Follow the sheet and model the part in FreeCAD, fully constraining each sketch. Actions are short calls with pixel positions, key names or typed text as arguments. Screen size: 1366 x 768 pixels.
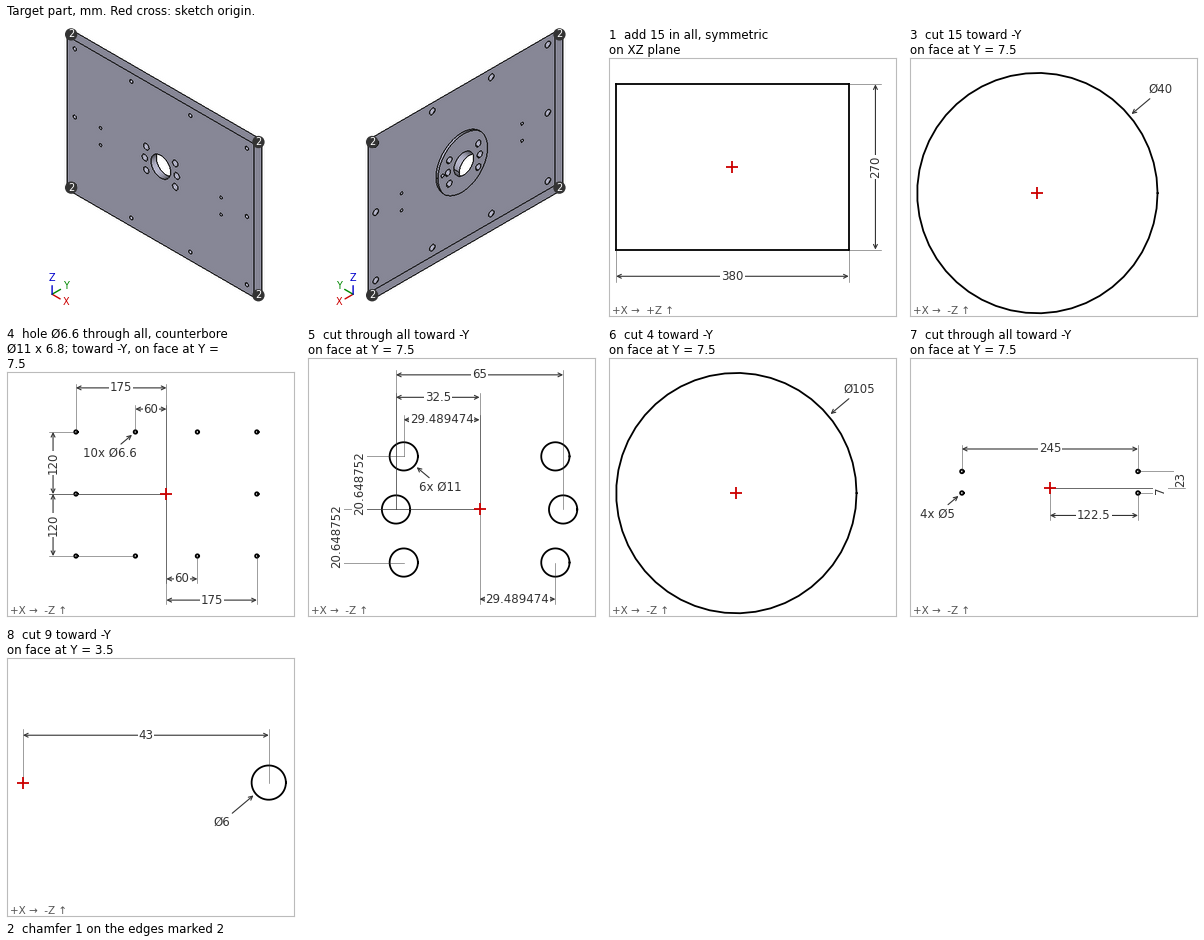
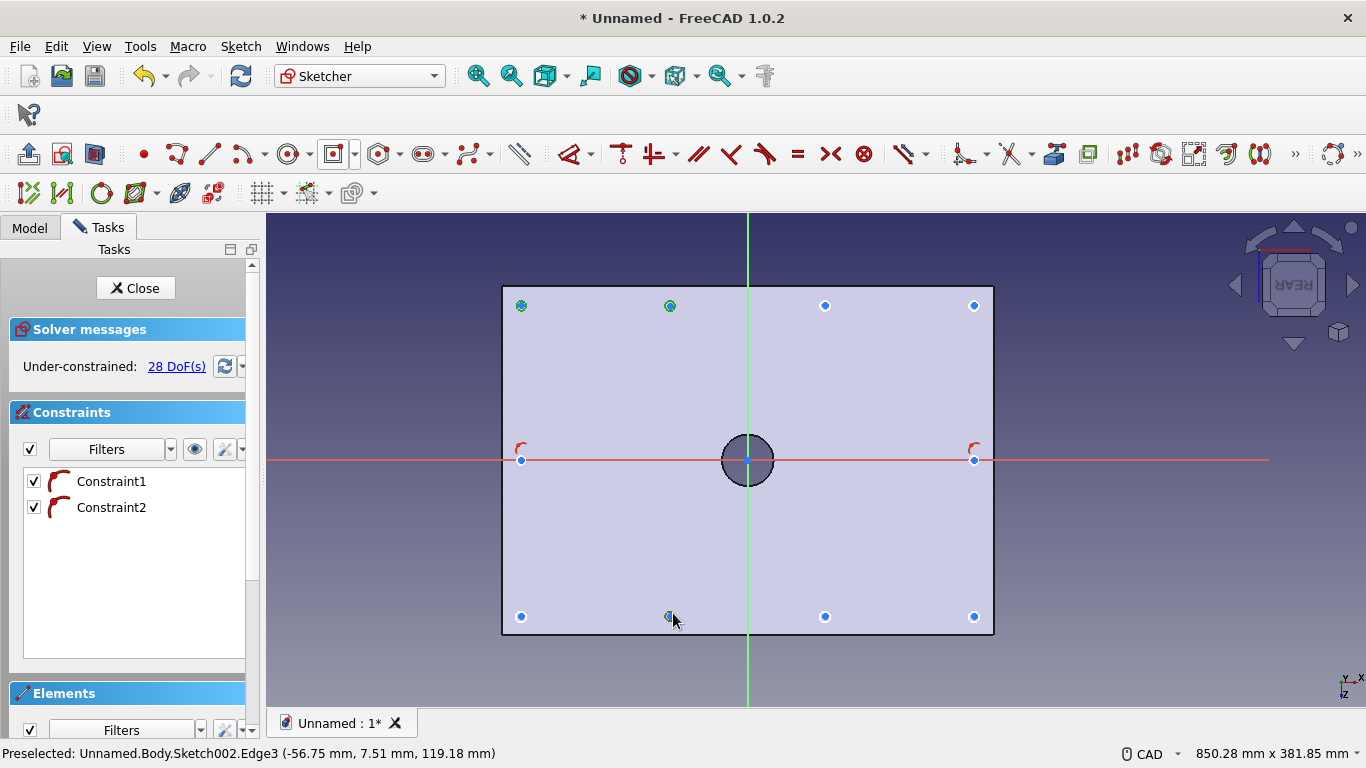
scroll(524, 457, up, 8)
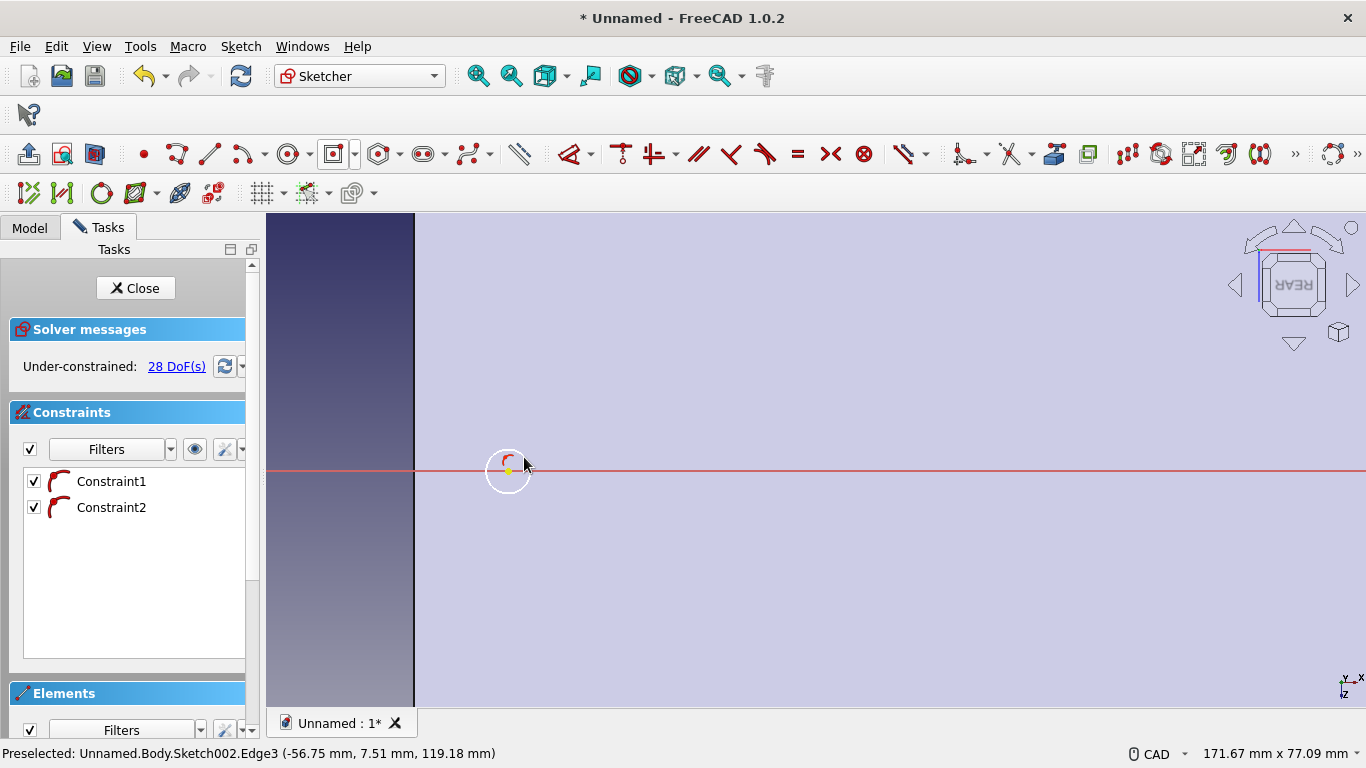
click(524, 456)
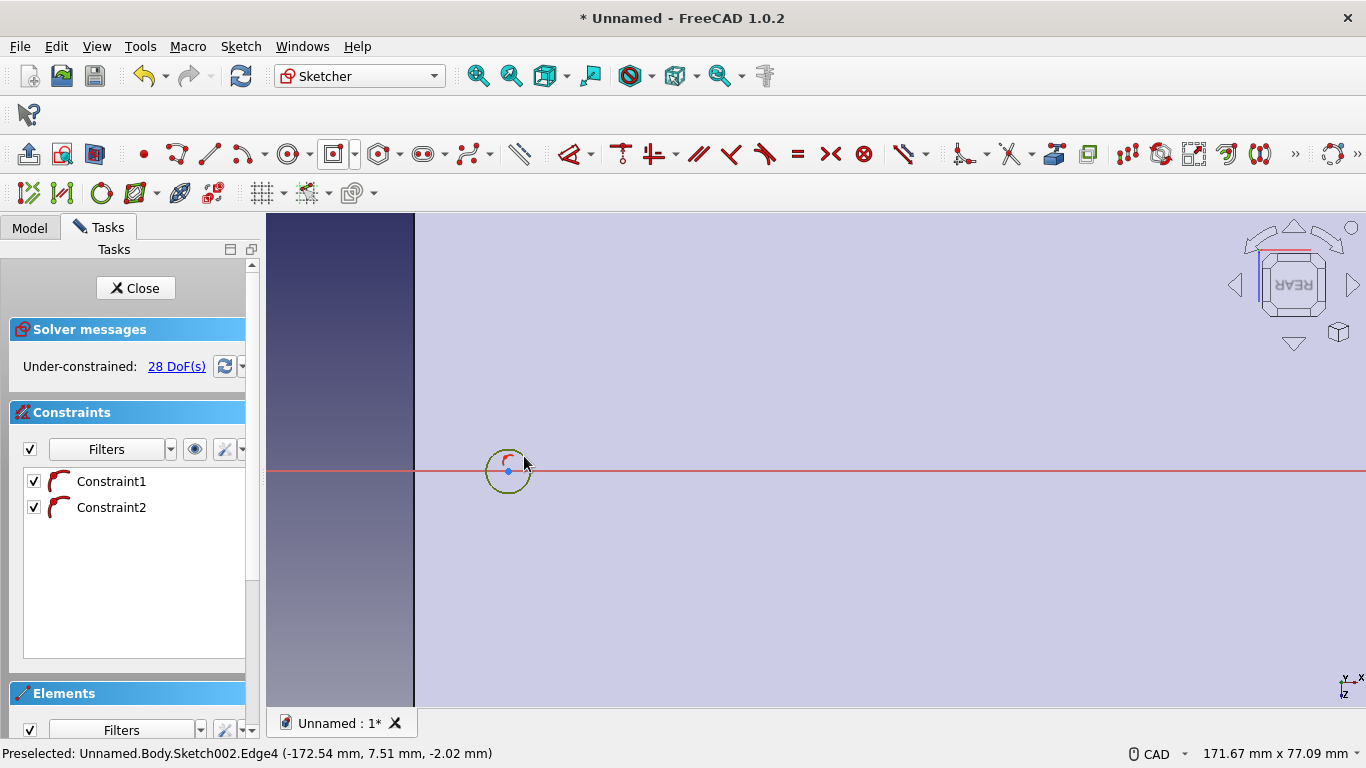
scroll(524, 457, down, 8)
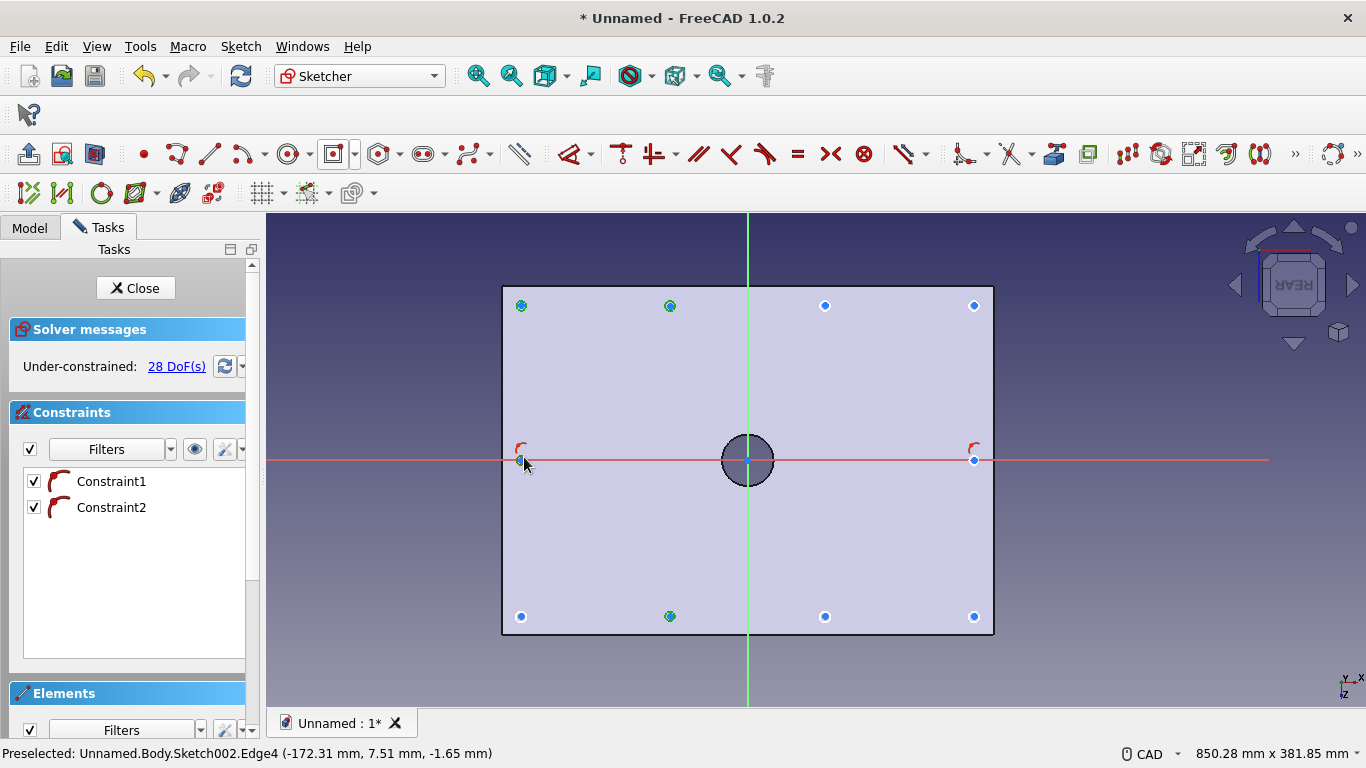
scroll(525, 613, up, 5)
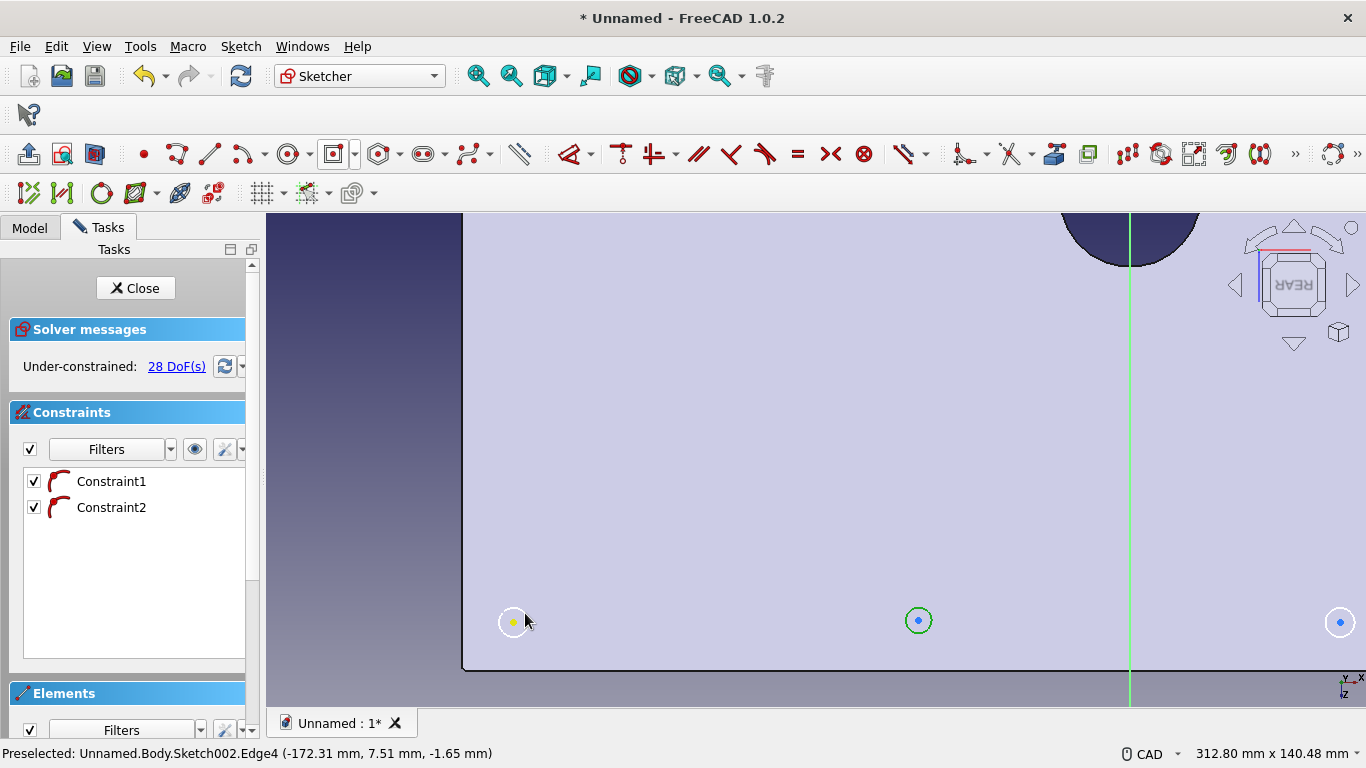
click(524, 612)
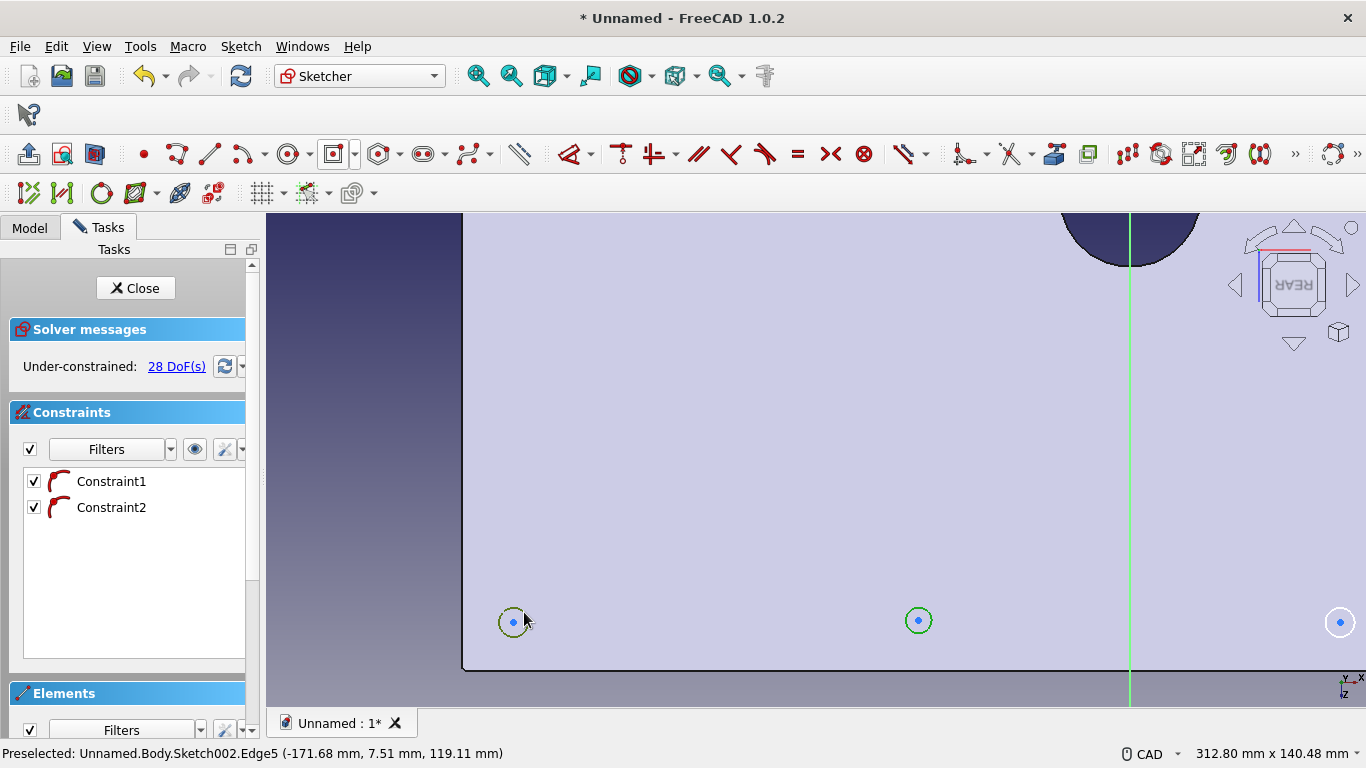
scroll(525, 613, down, 5)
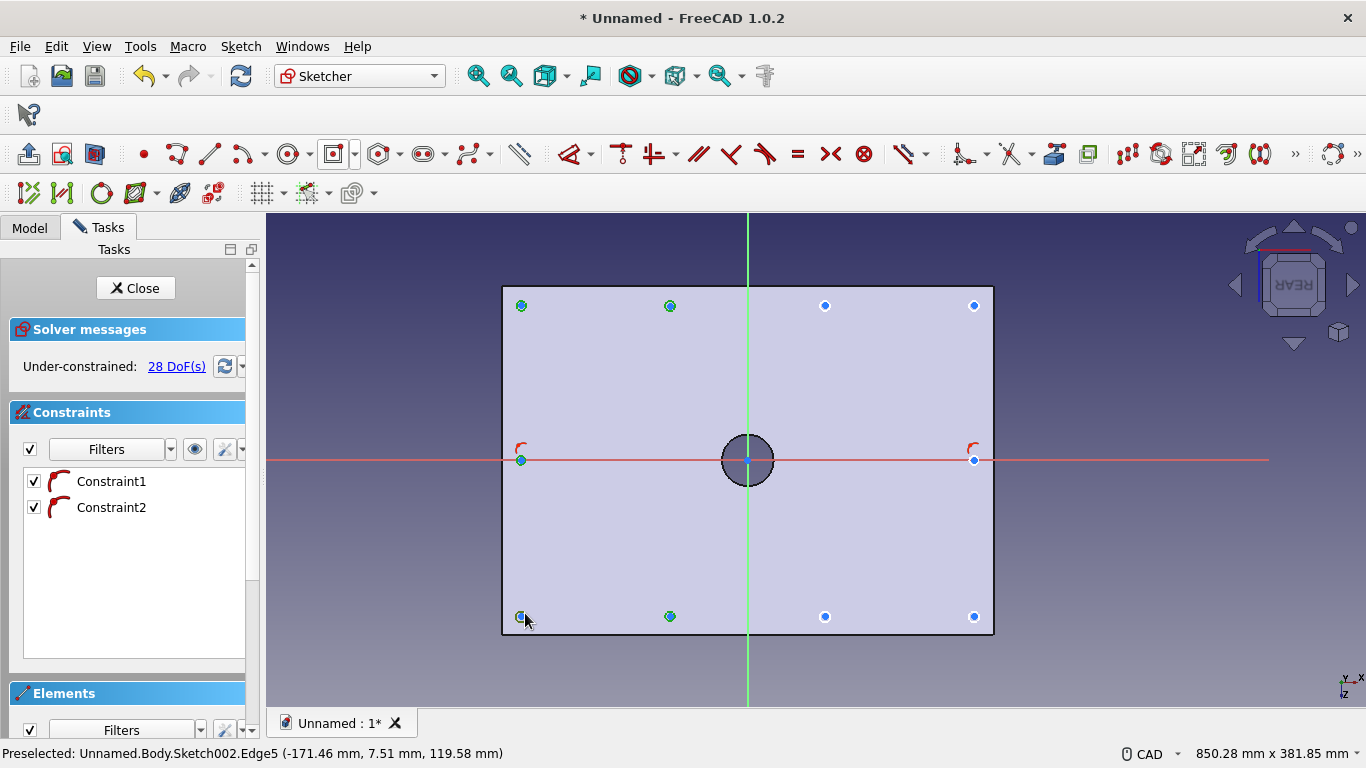
scroll(978, 613, up, 5)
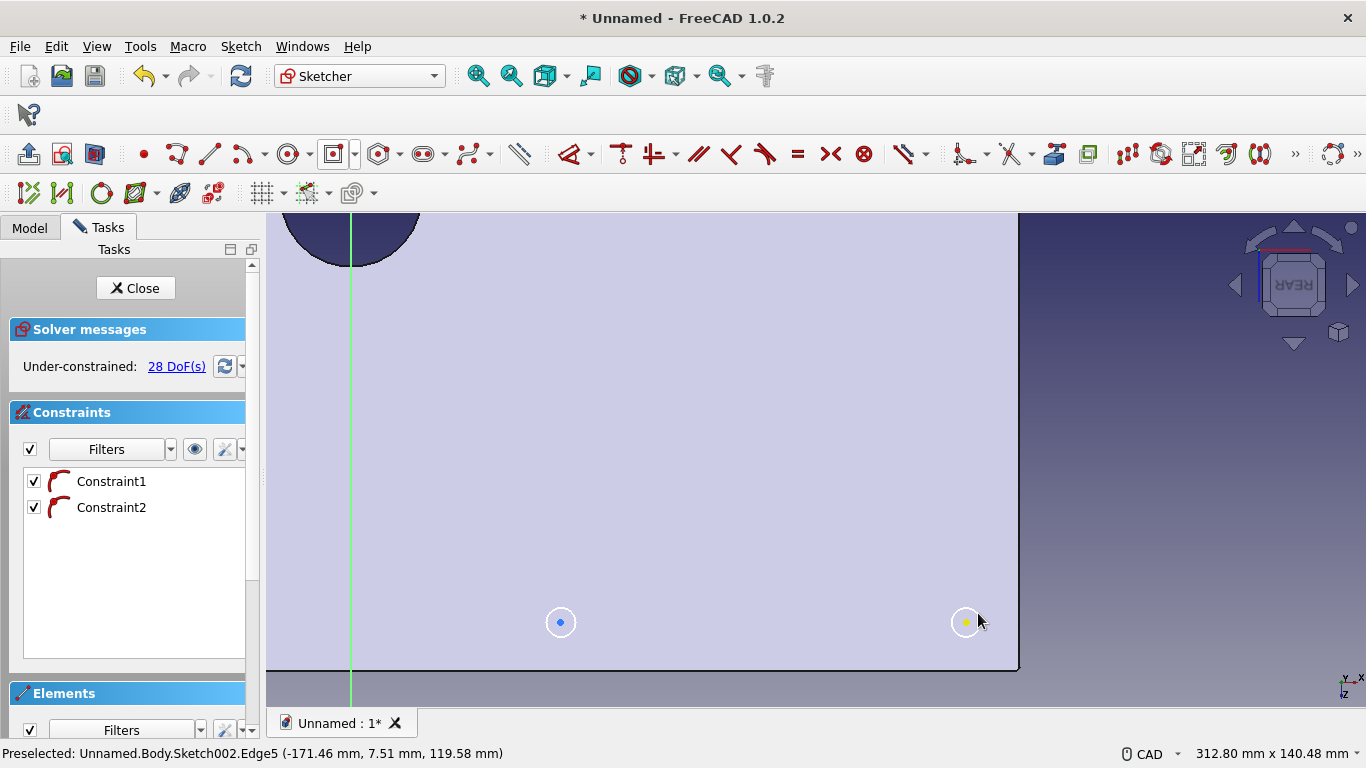
click(976, 612)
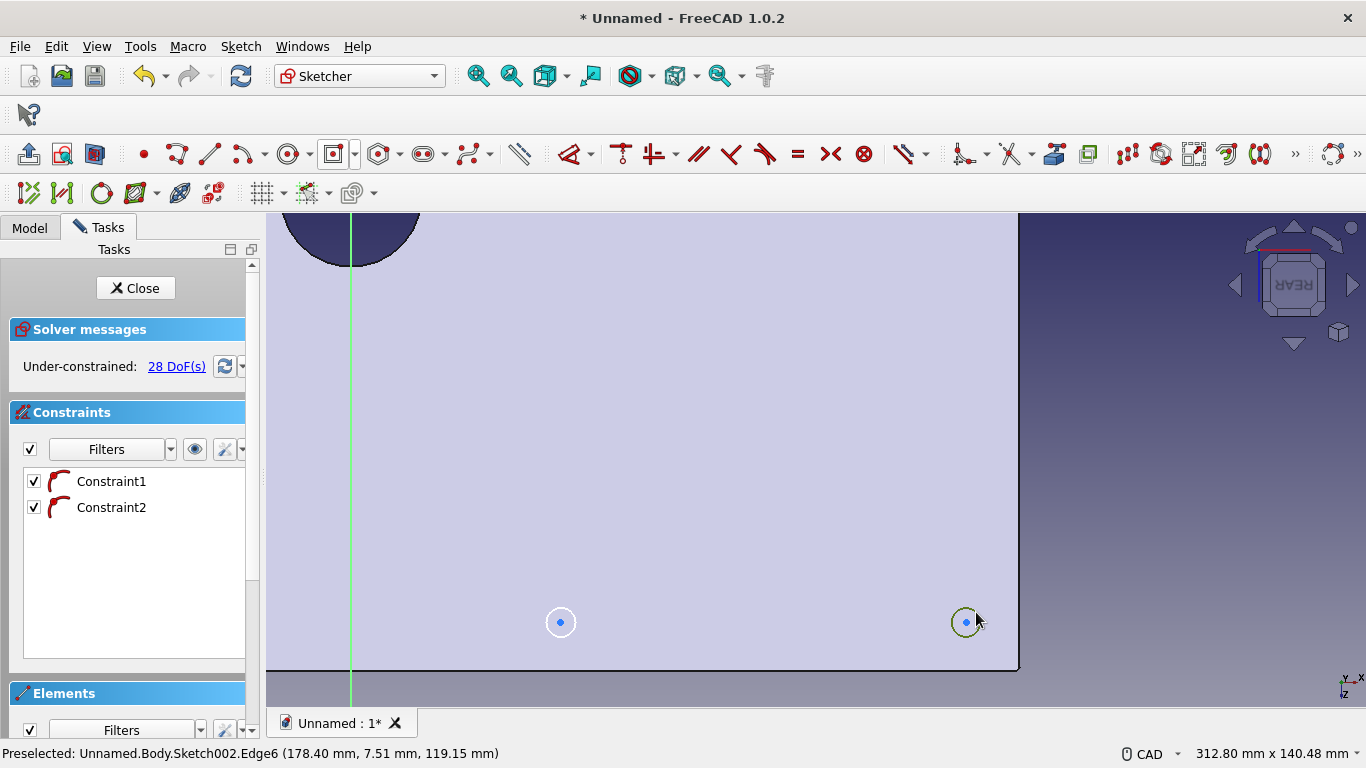
scroll(978, 613, down, 5)